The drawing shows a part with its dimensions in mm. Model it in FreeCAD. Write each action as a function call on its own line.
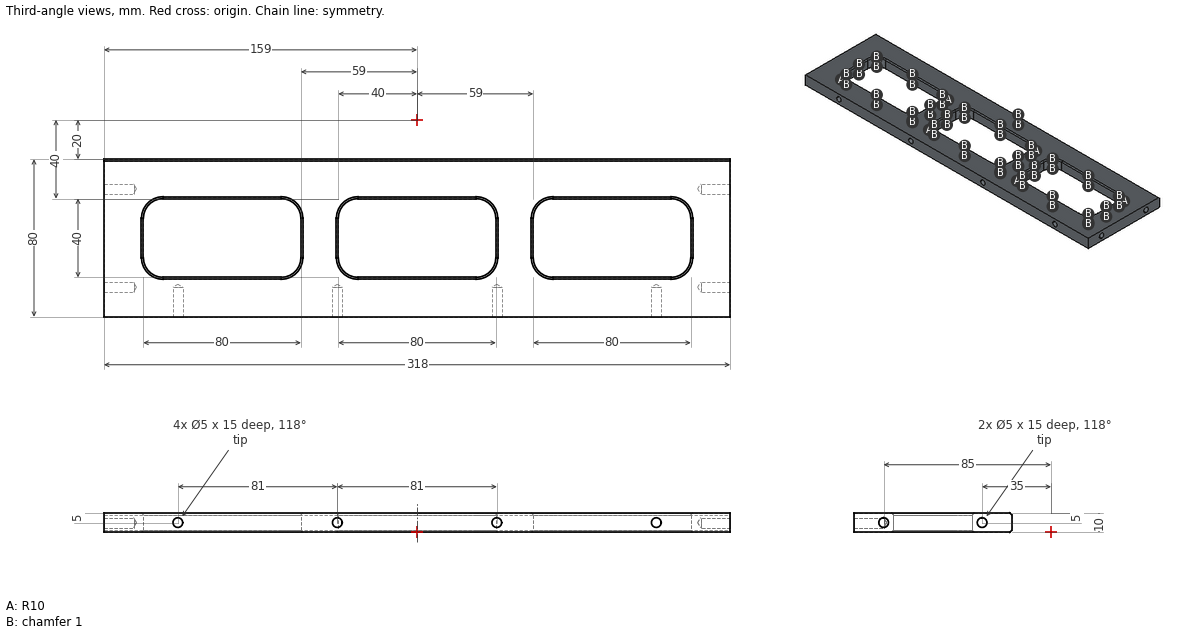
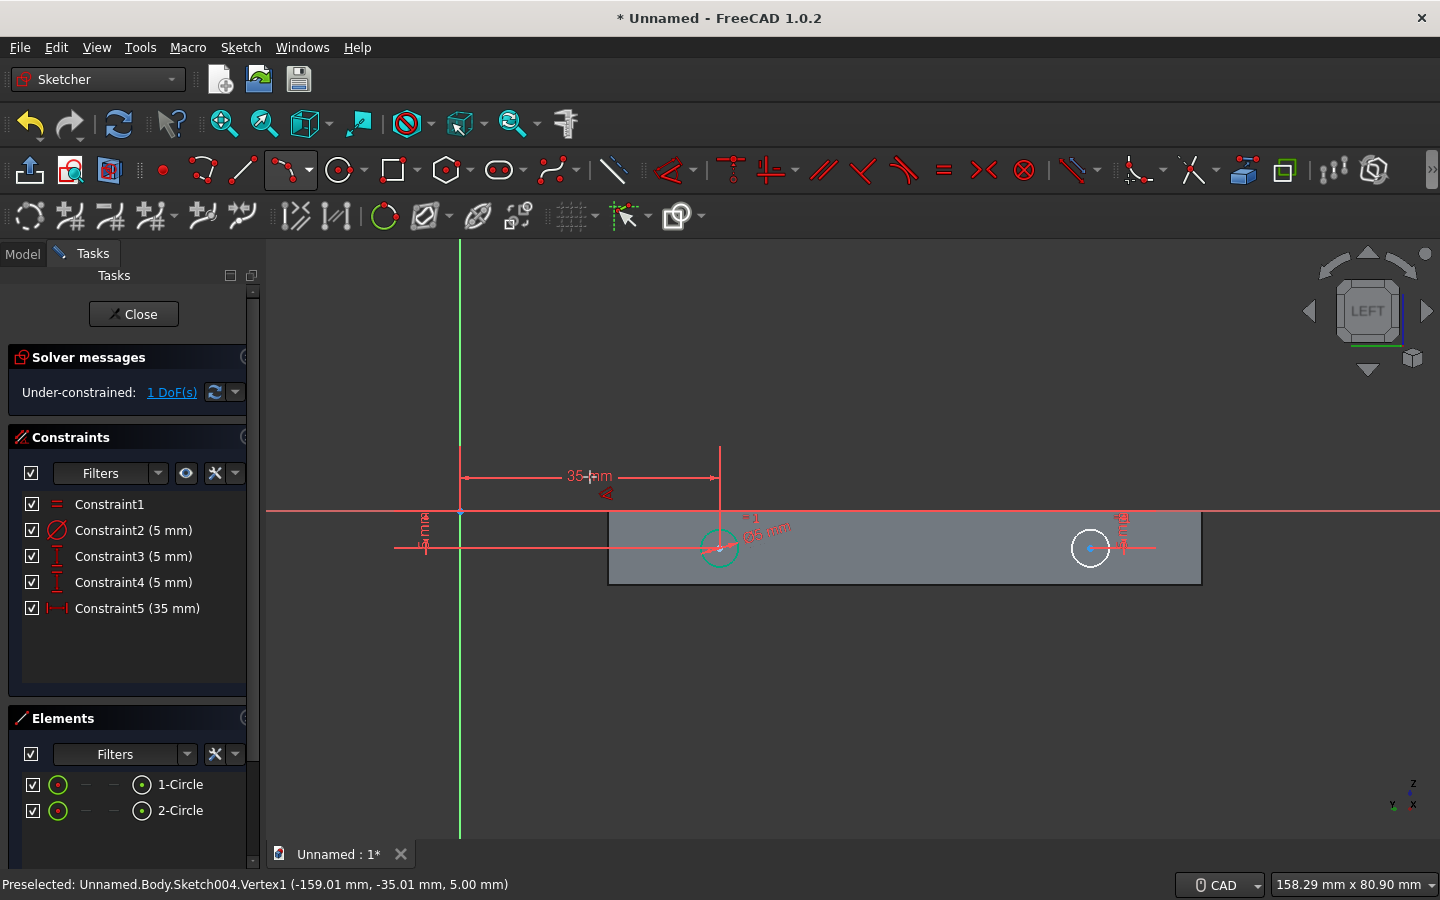
click(1090, 548)
click(775, 477)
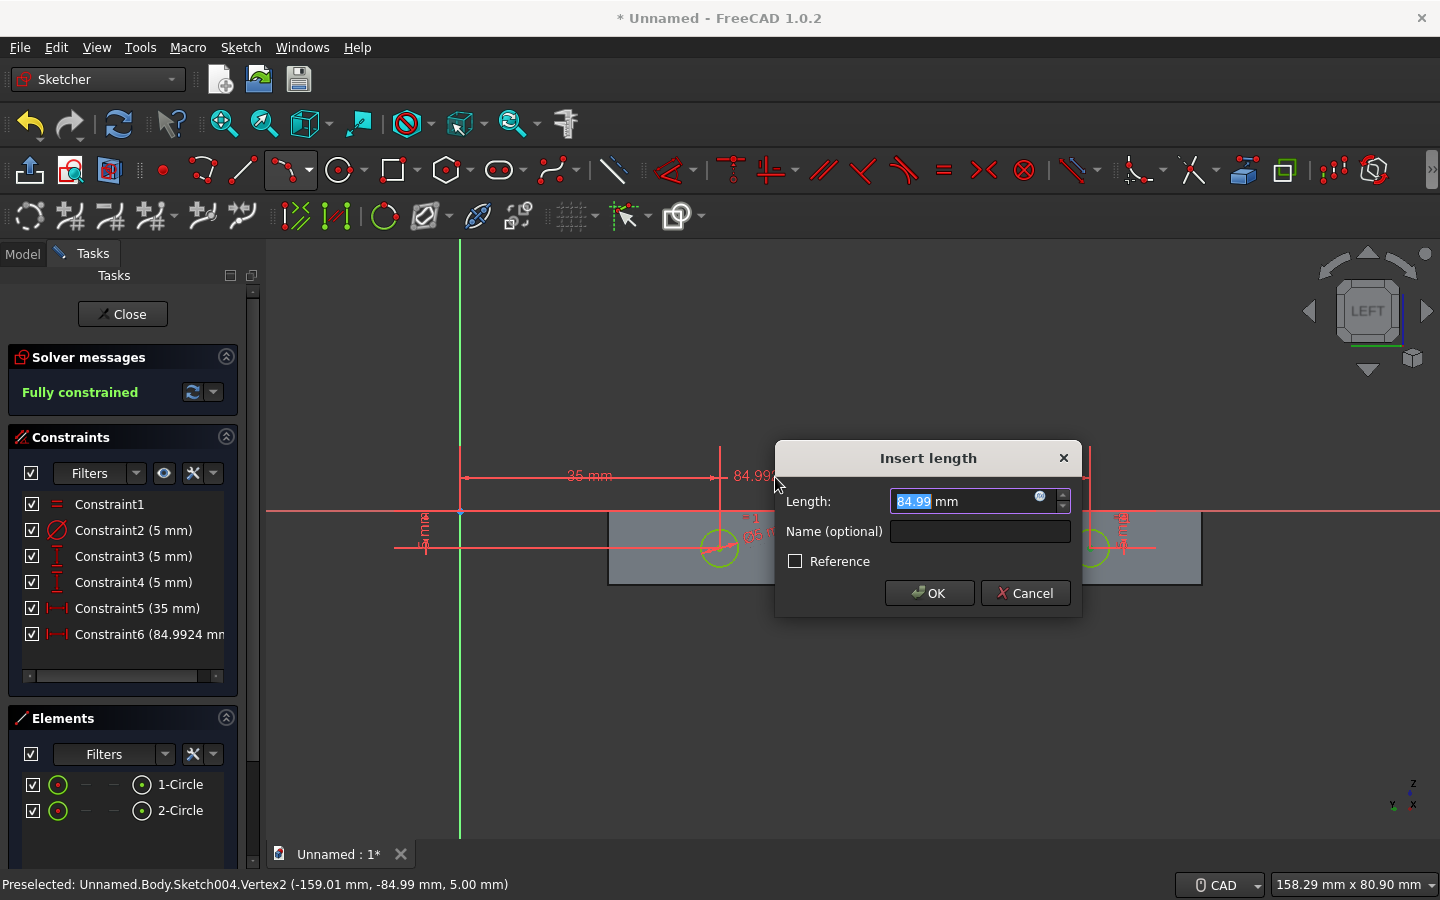
text(85)
key(Return)
key(Escape)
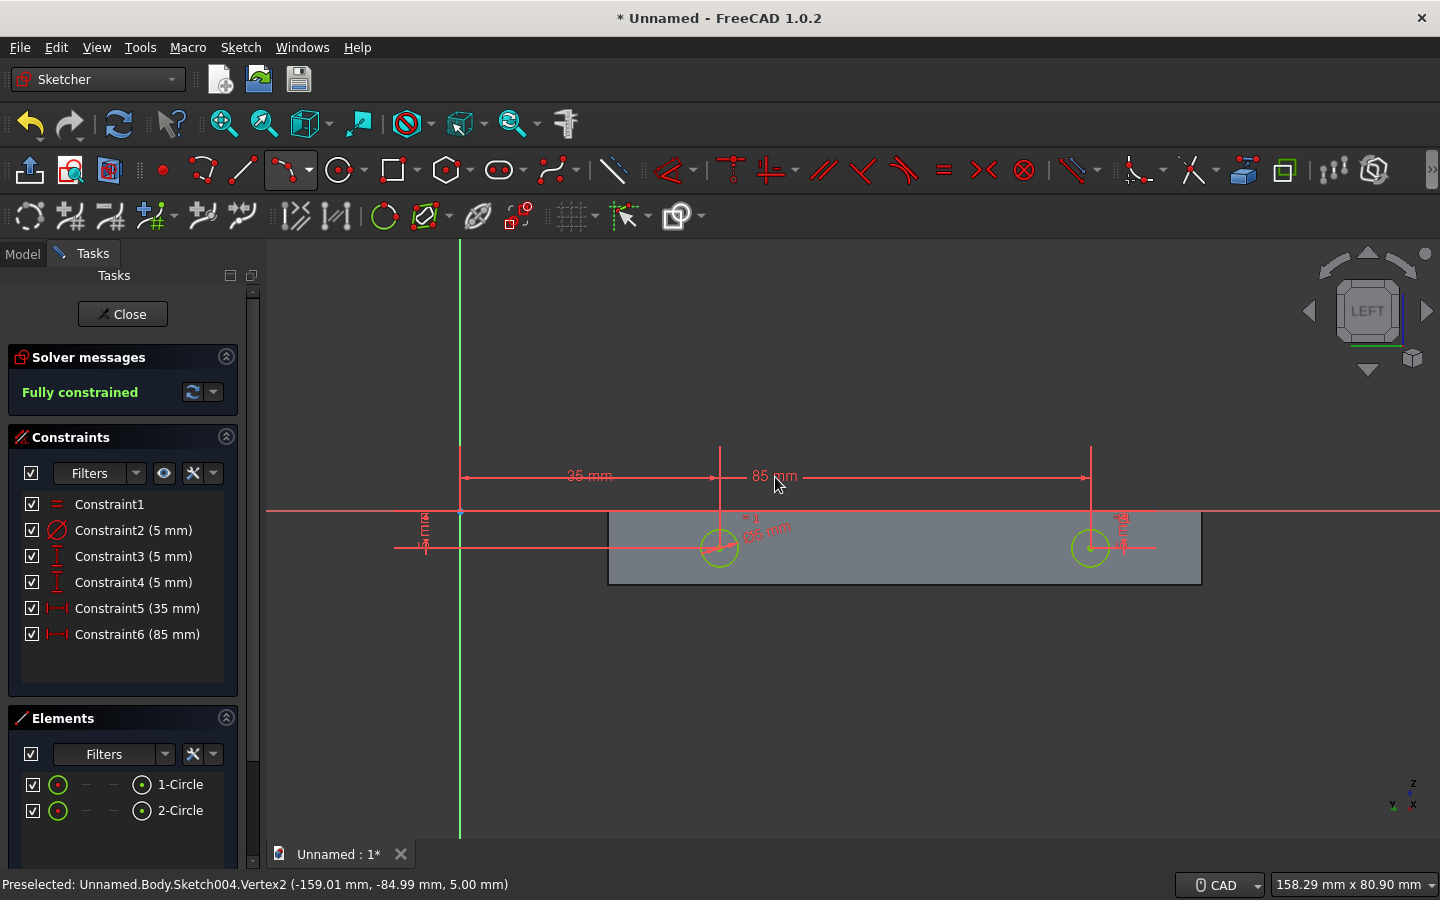
click(123, 314)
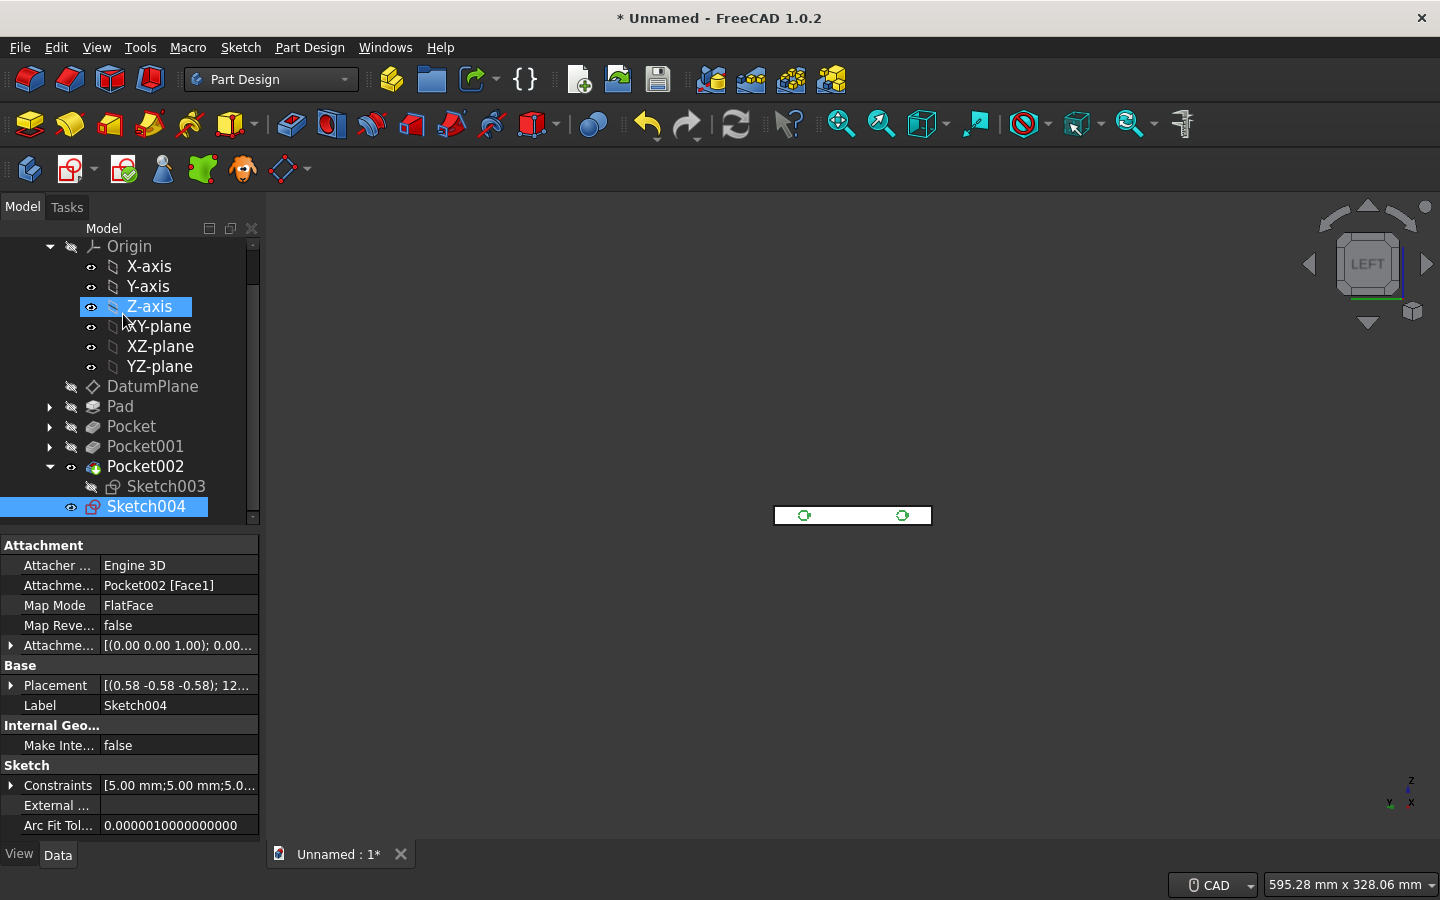
click(332, 124)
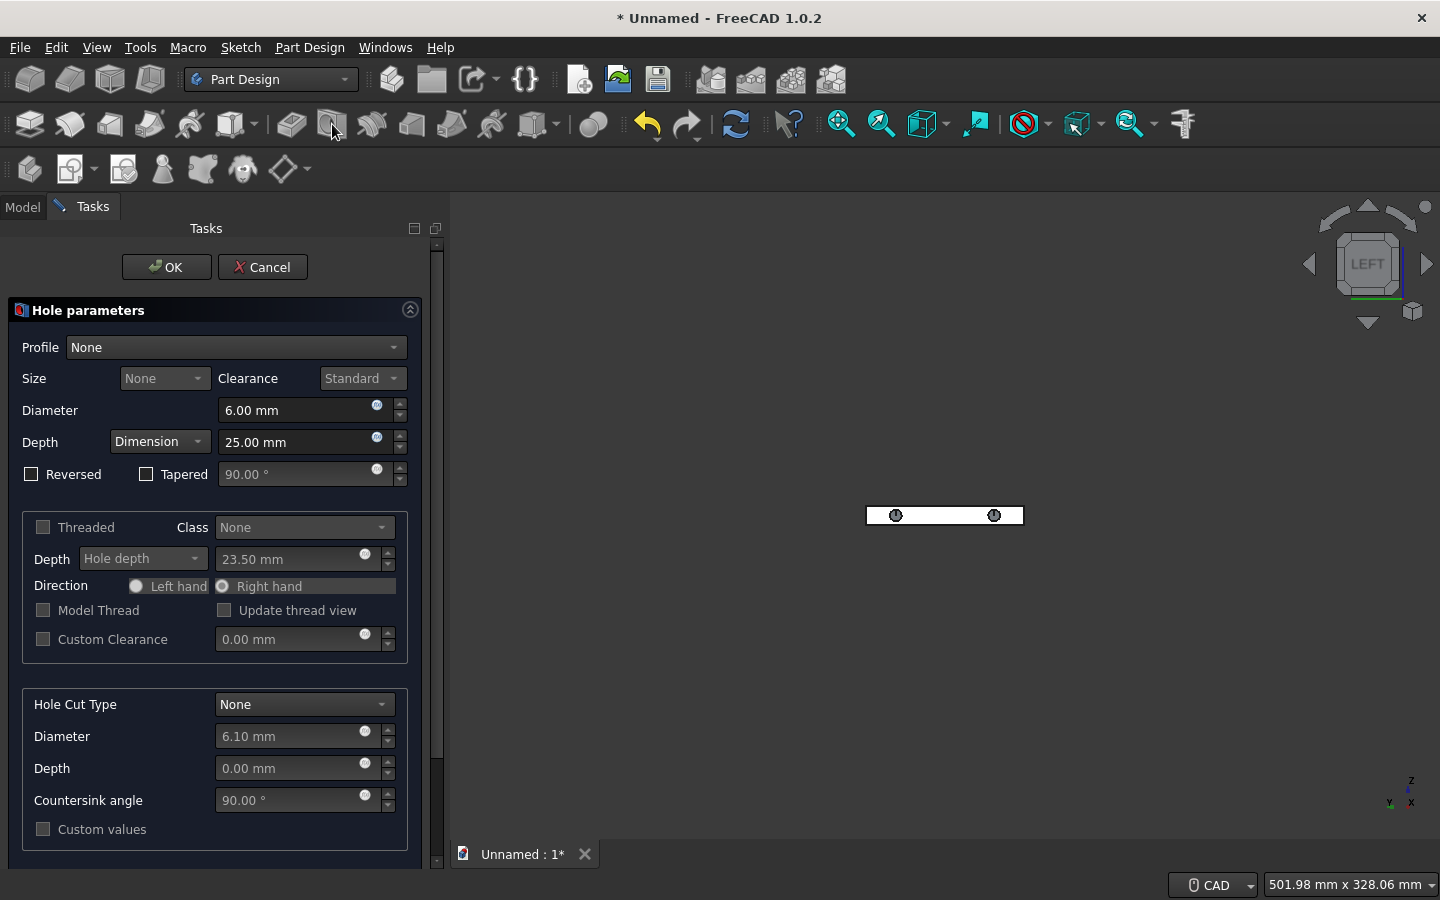
triple_click(305, 410)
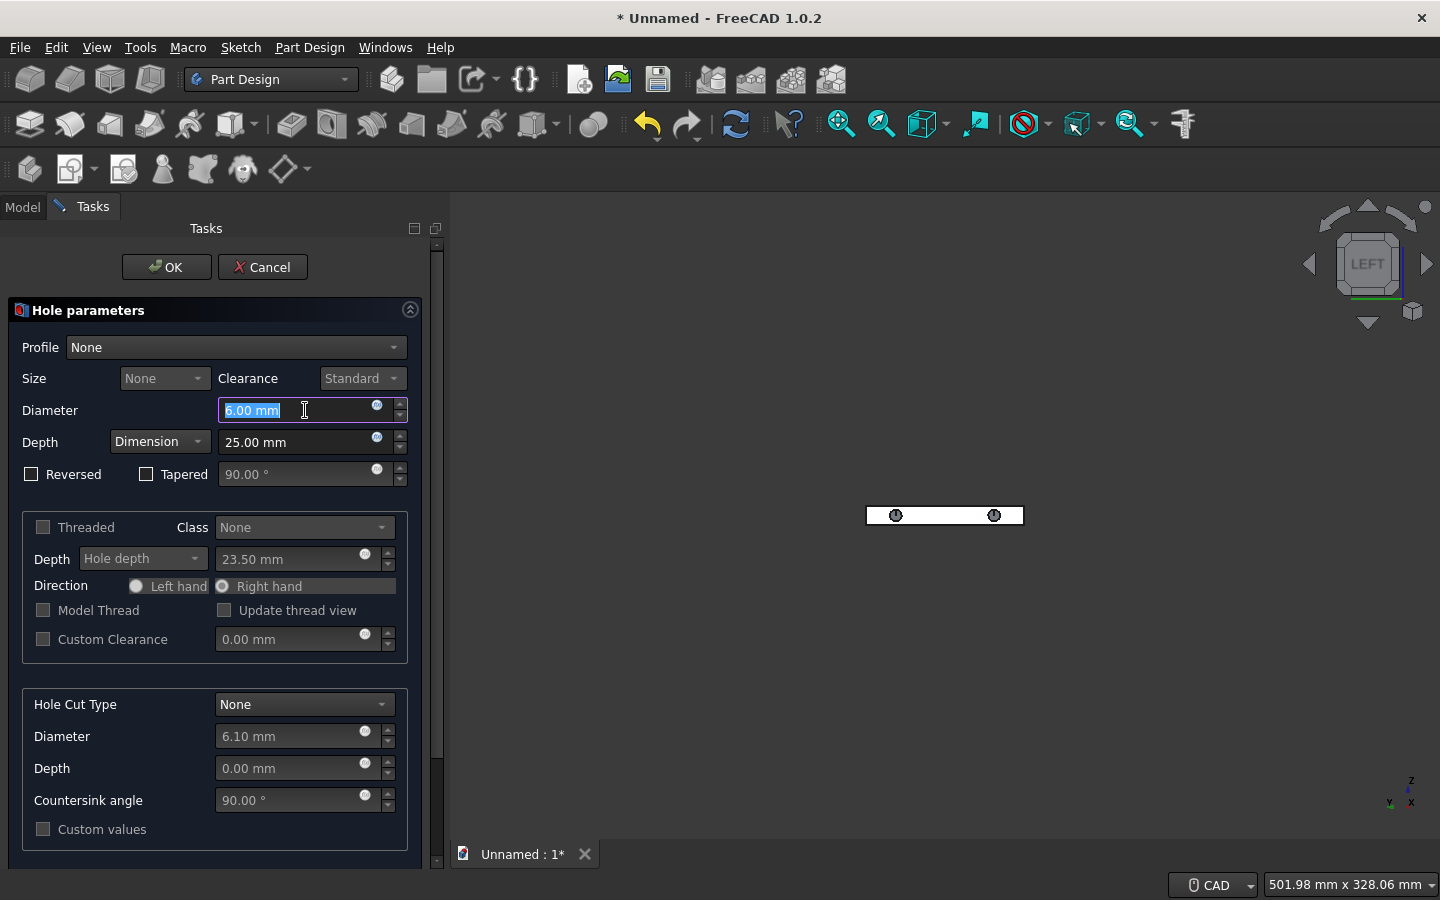
text(5)
key(Tab)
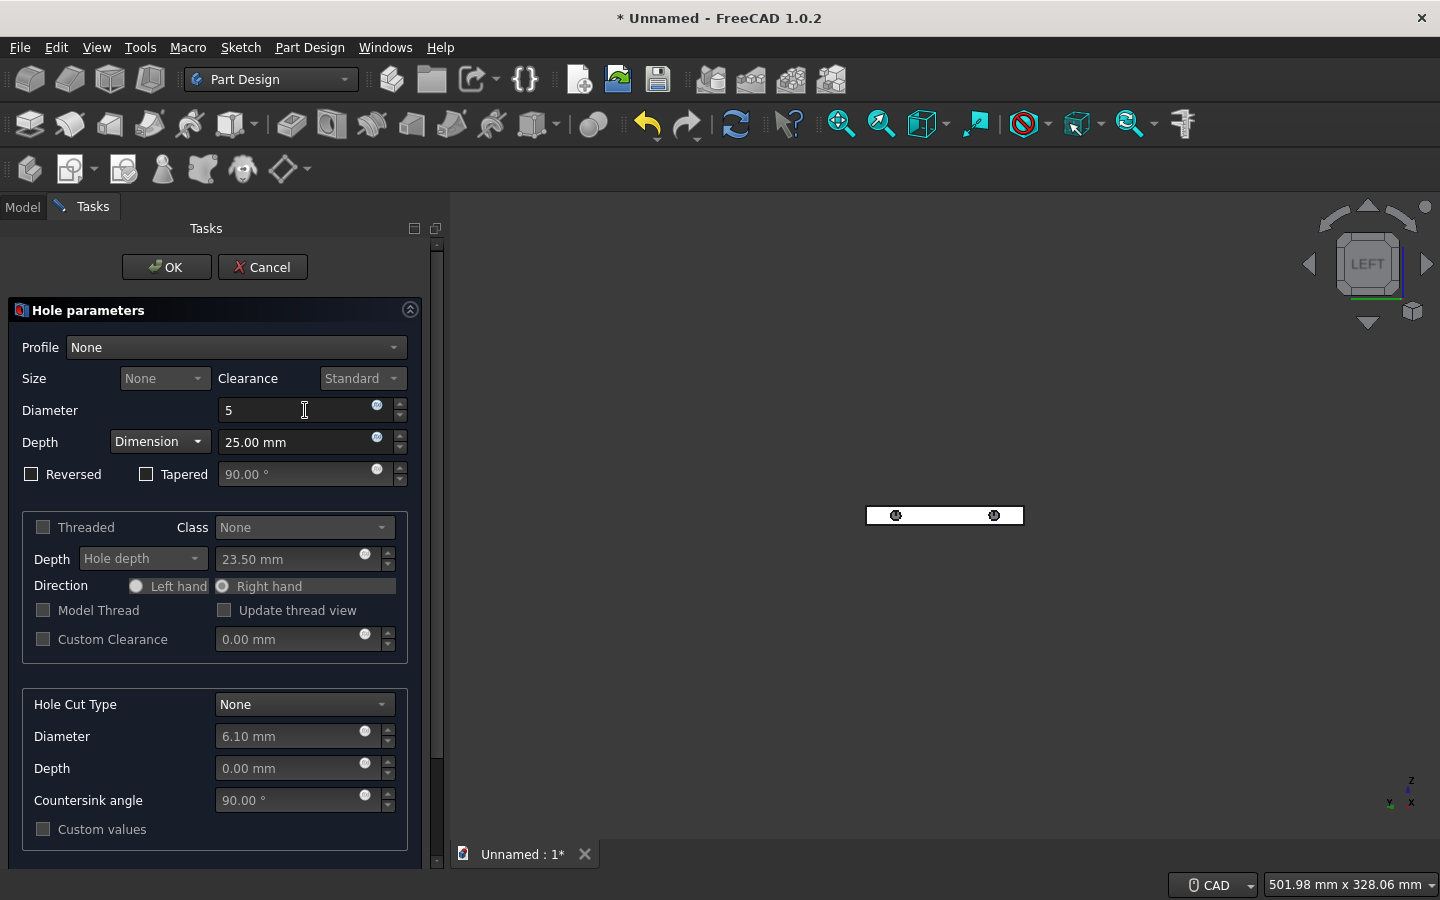
triple_click(305, 442)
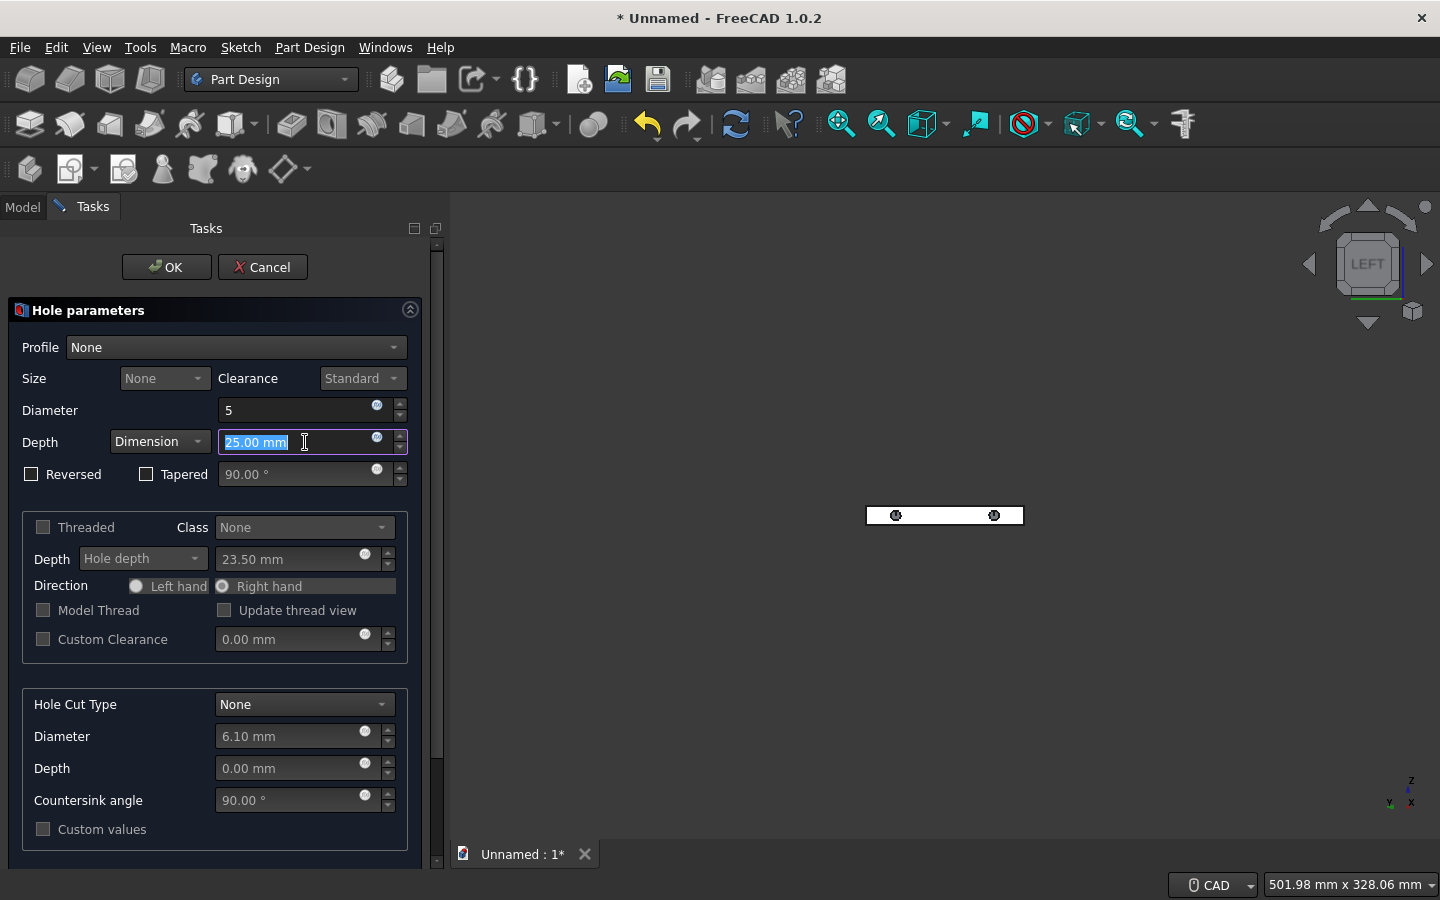
text(15)
key(Tab)